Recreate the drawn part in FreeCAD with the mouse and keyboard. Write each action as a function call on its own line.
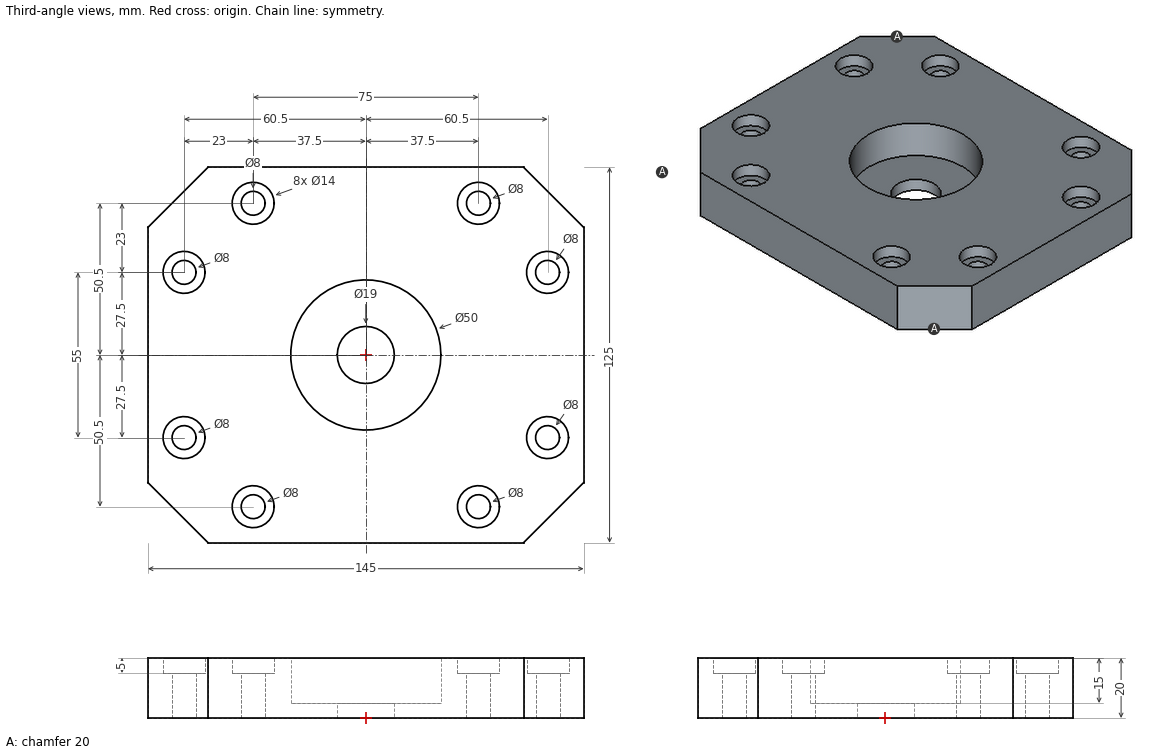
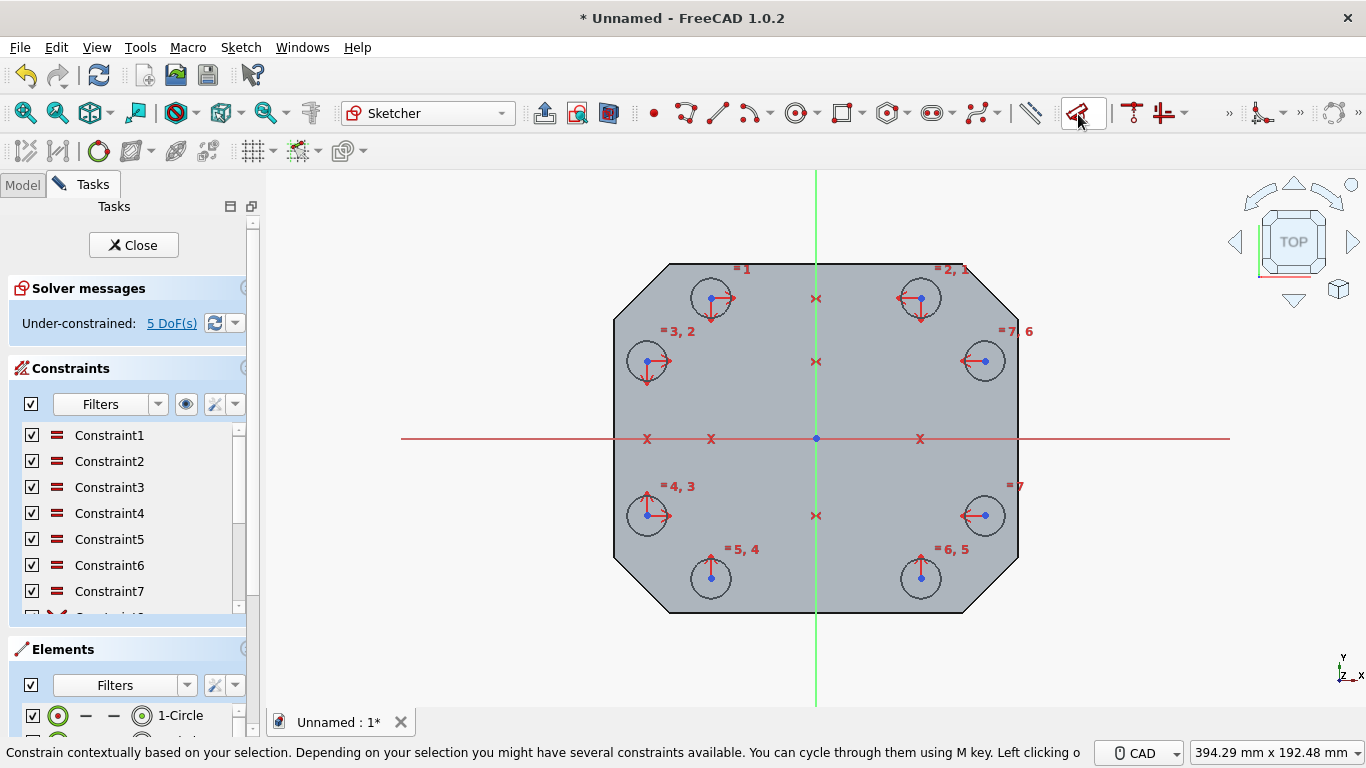
click(725, 284)
click(747, 261)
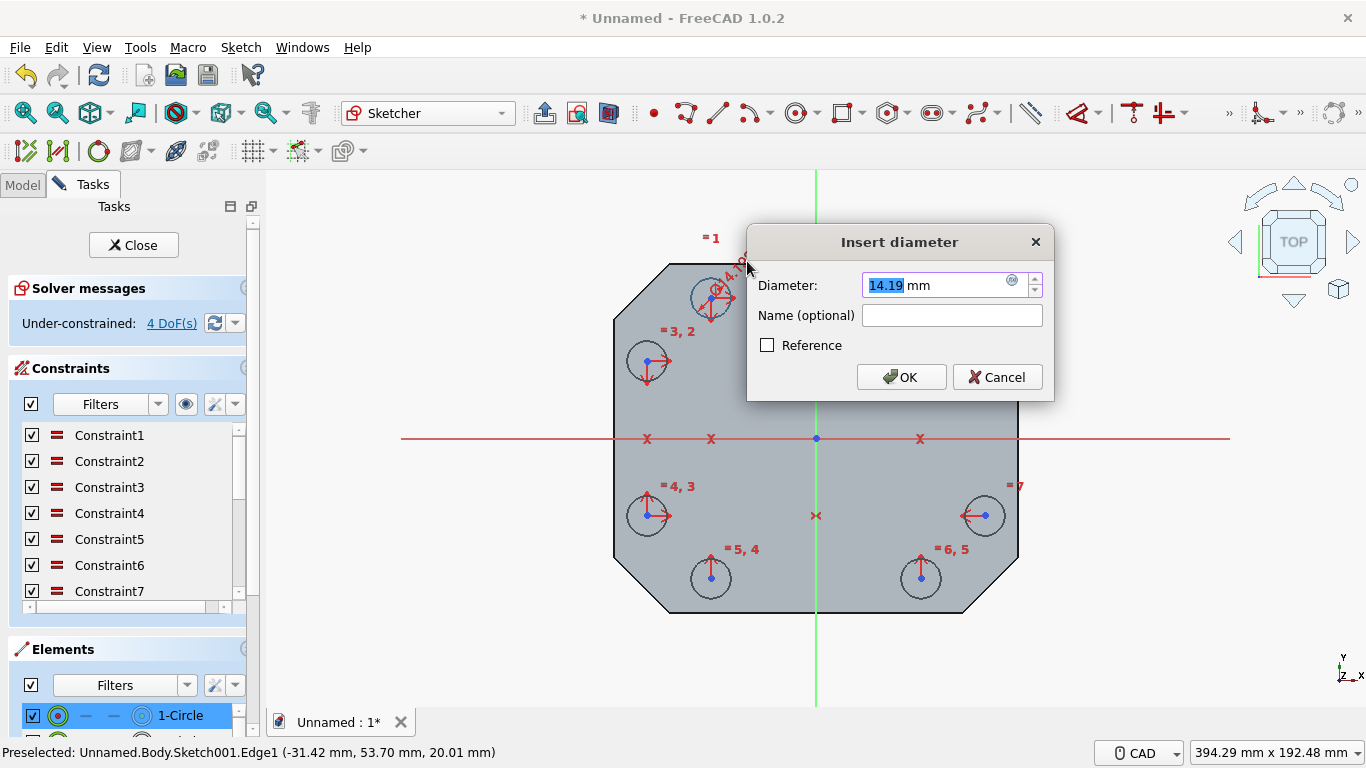
text(14)
key(Return)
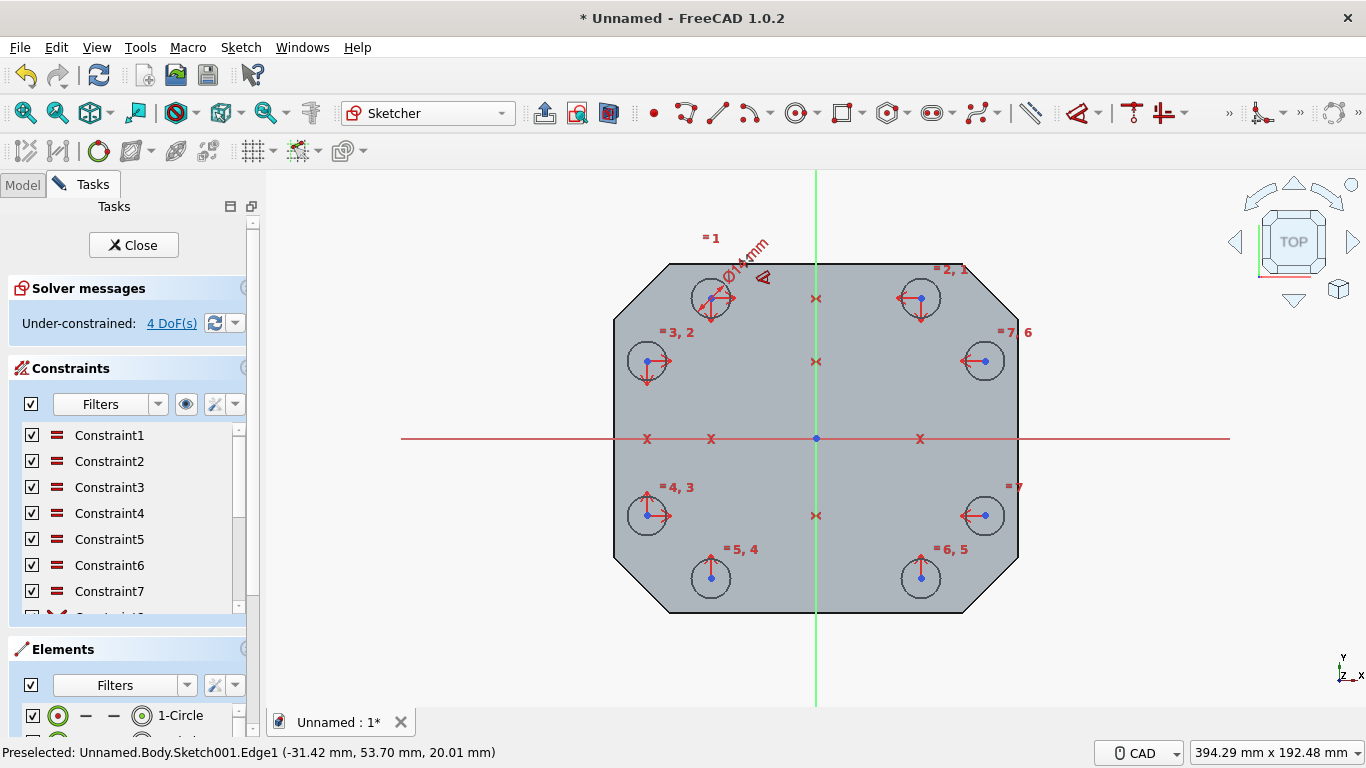
click(711, 298)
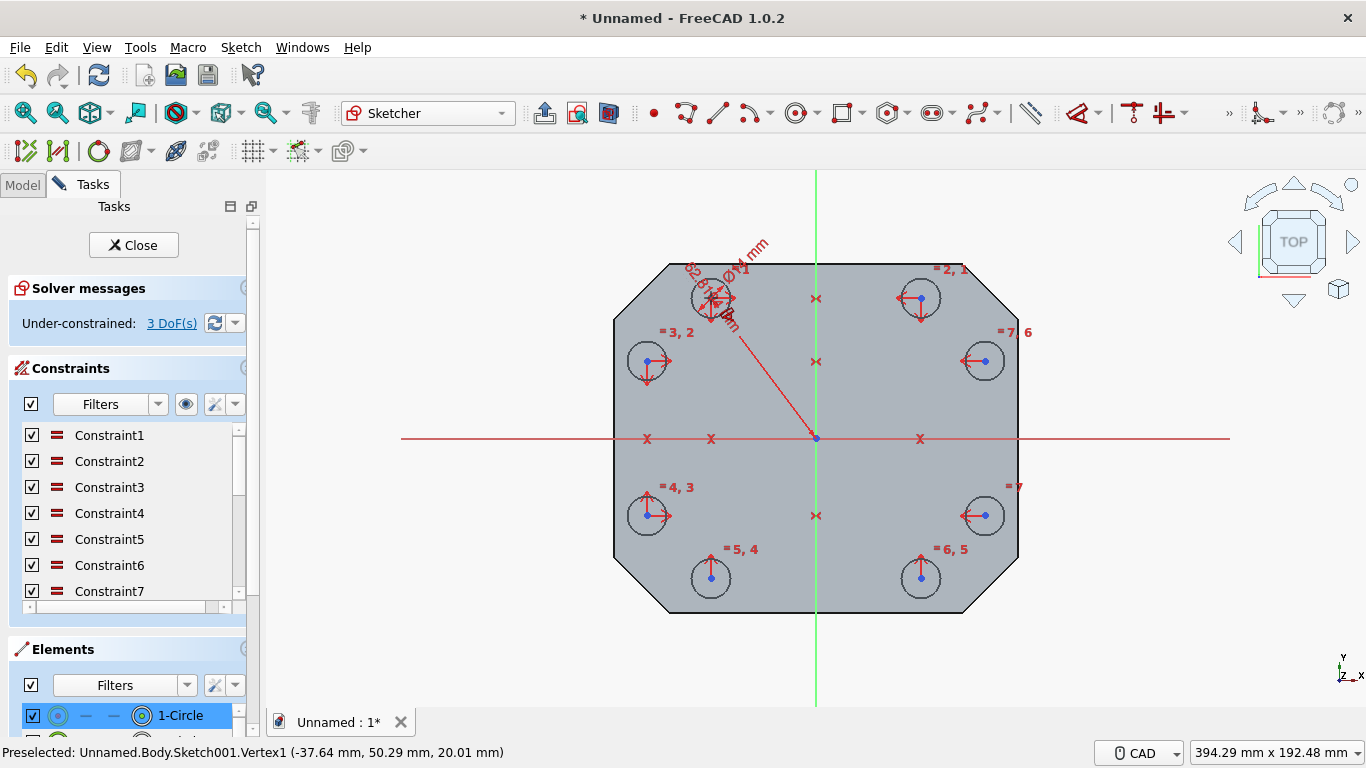
click(921, 298)
click(864, 264)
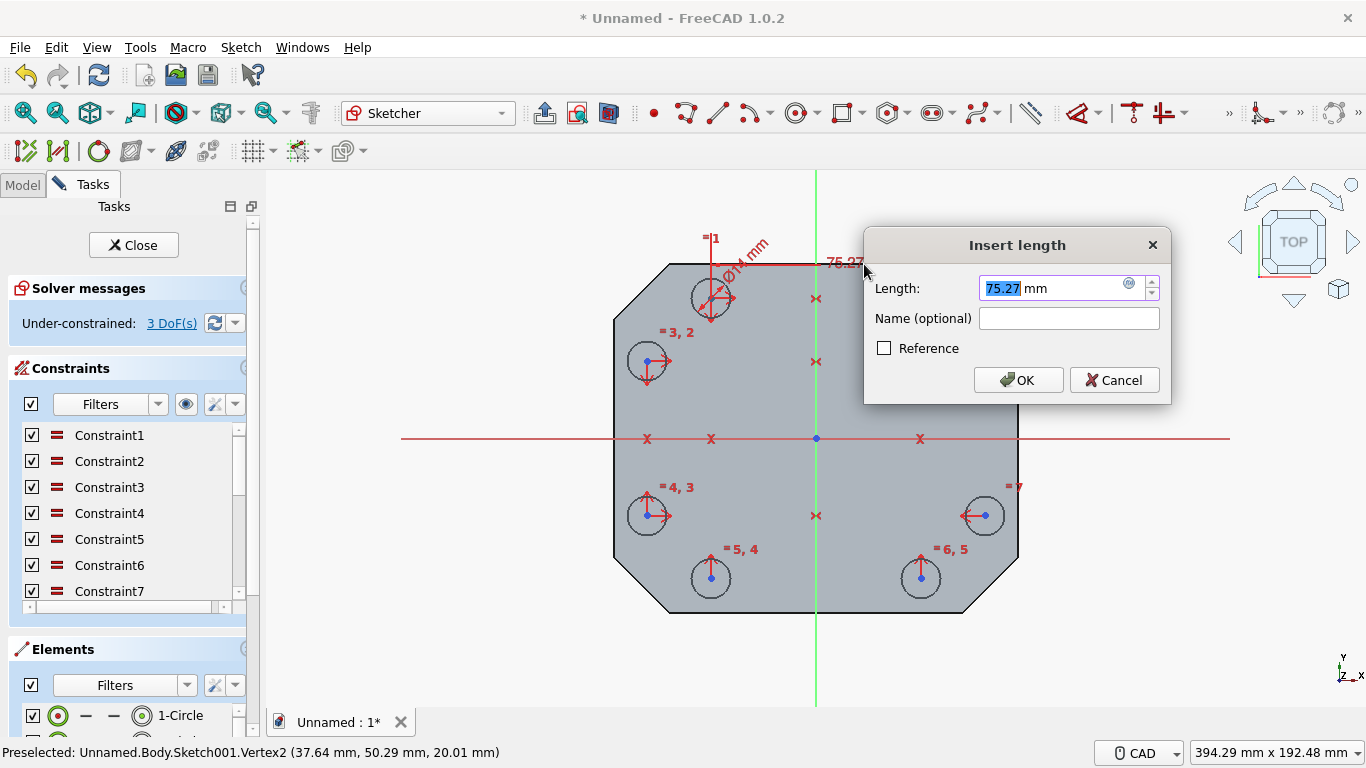
text(75)
key(Return)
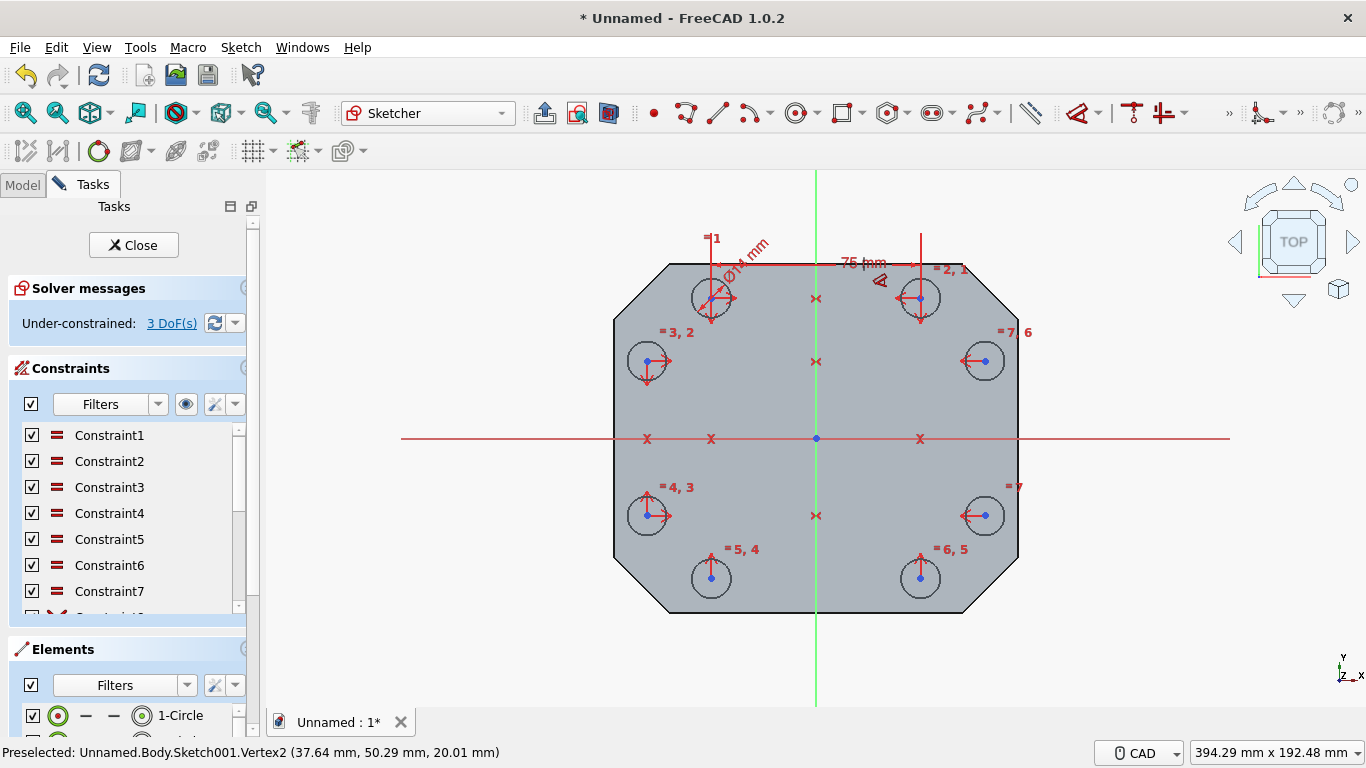
click(711, 298)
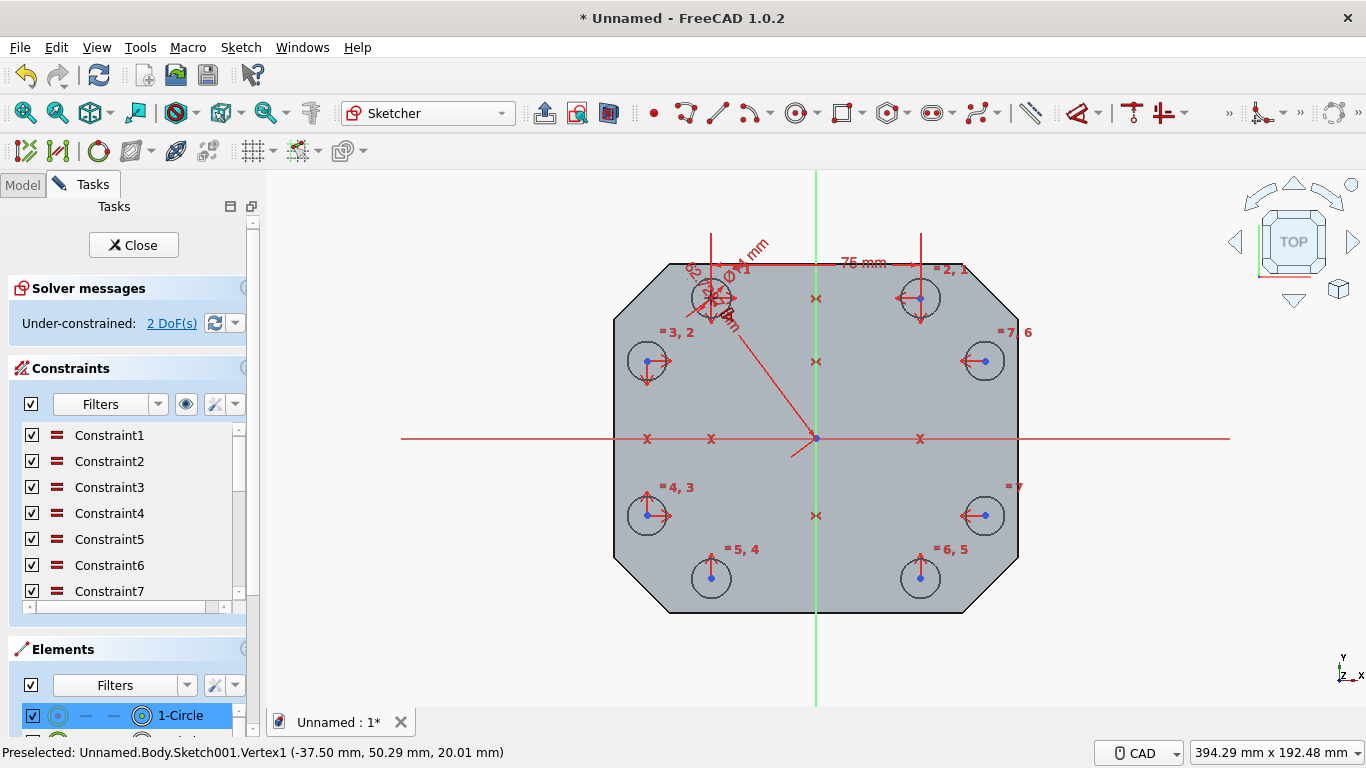
click(647, 361)
click(664, 264)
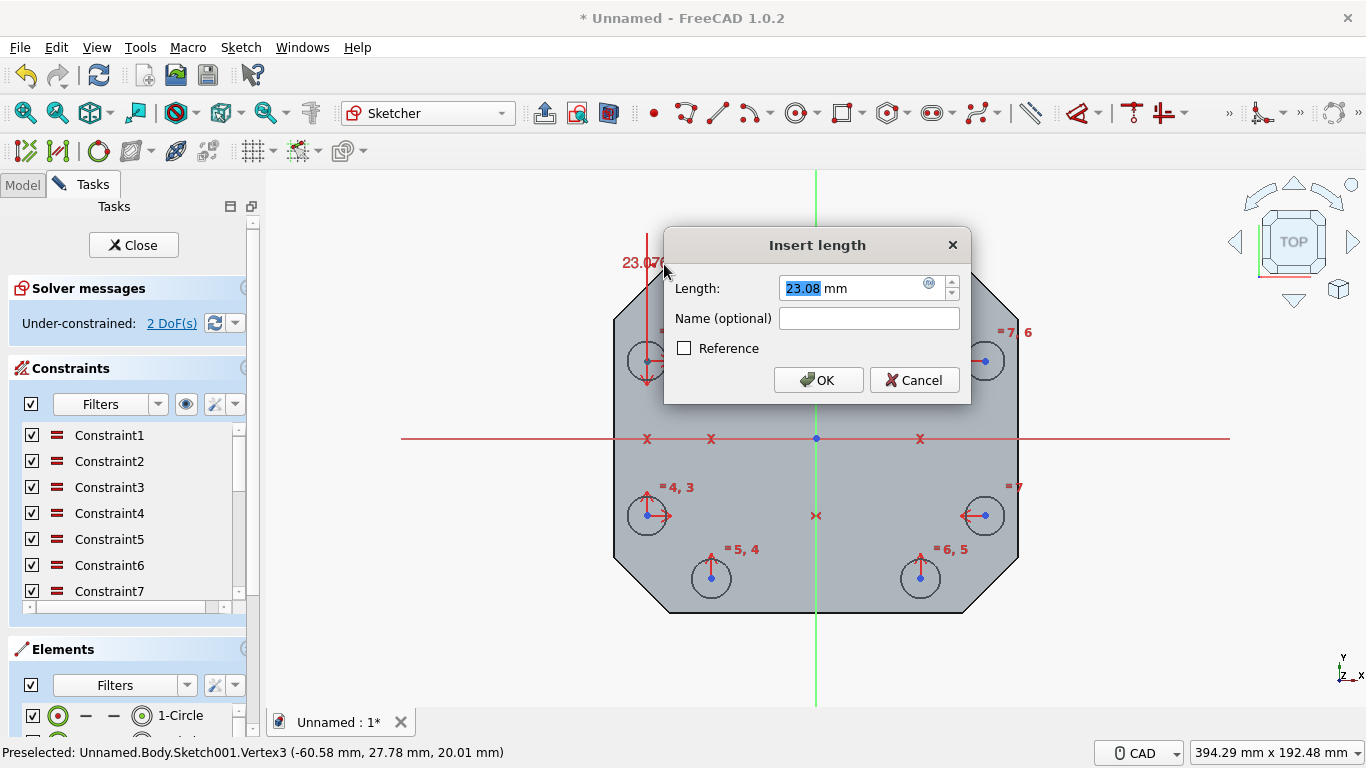
text(23)
key(Return)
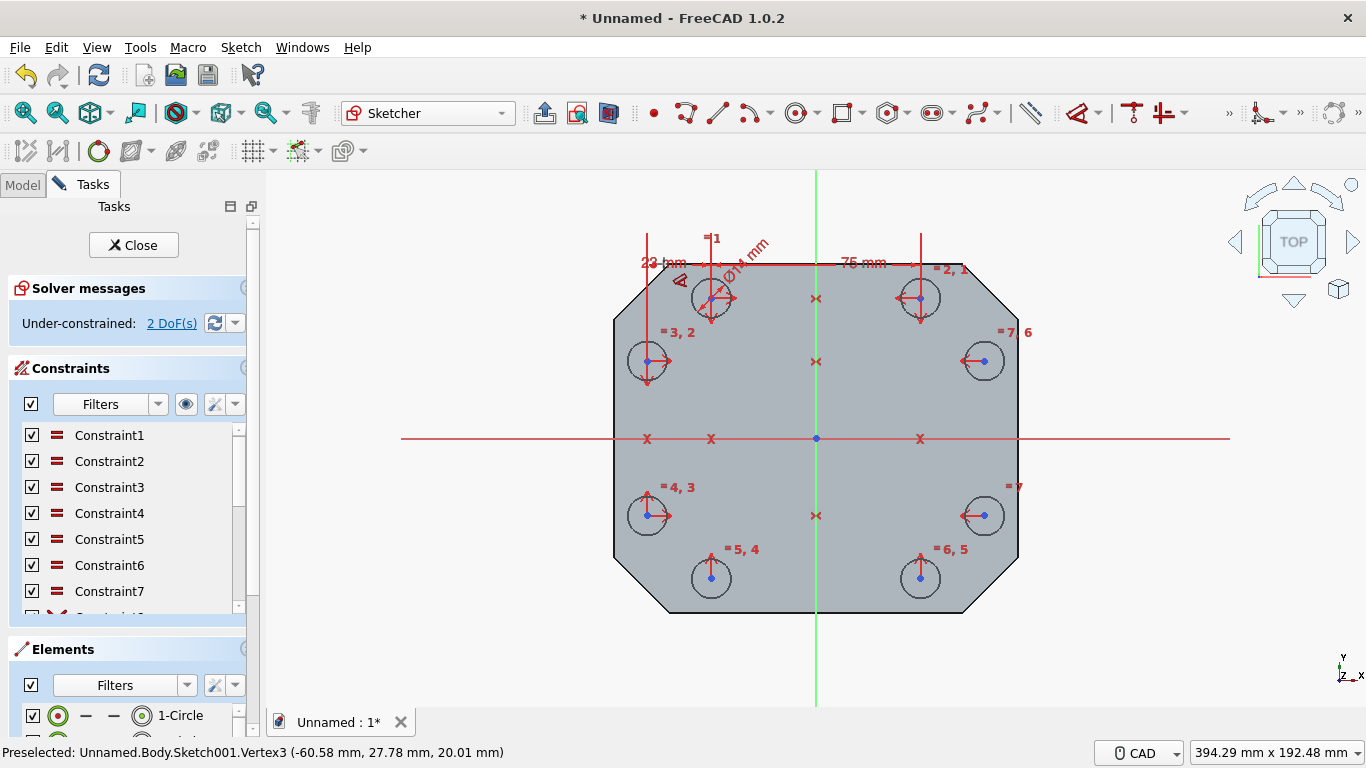
click(711, 298)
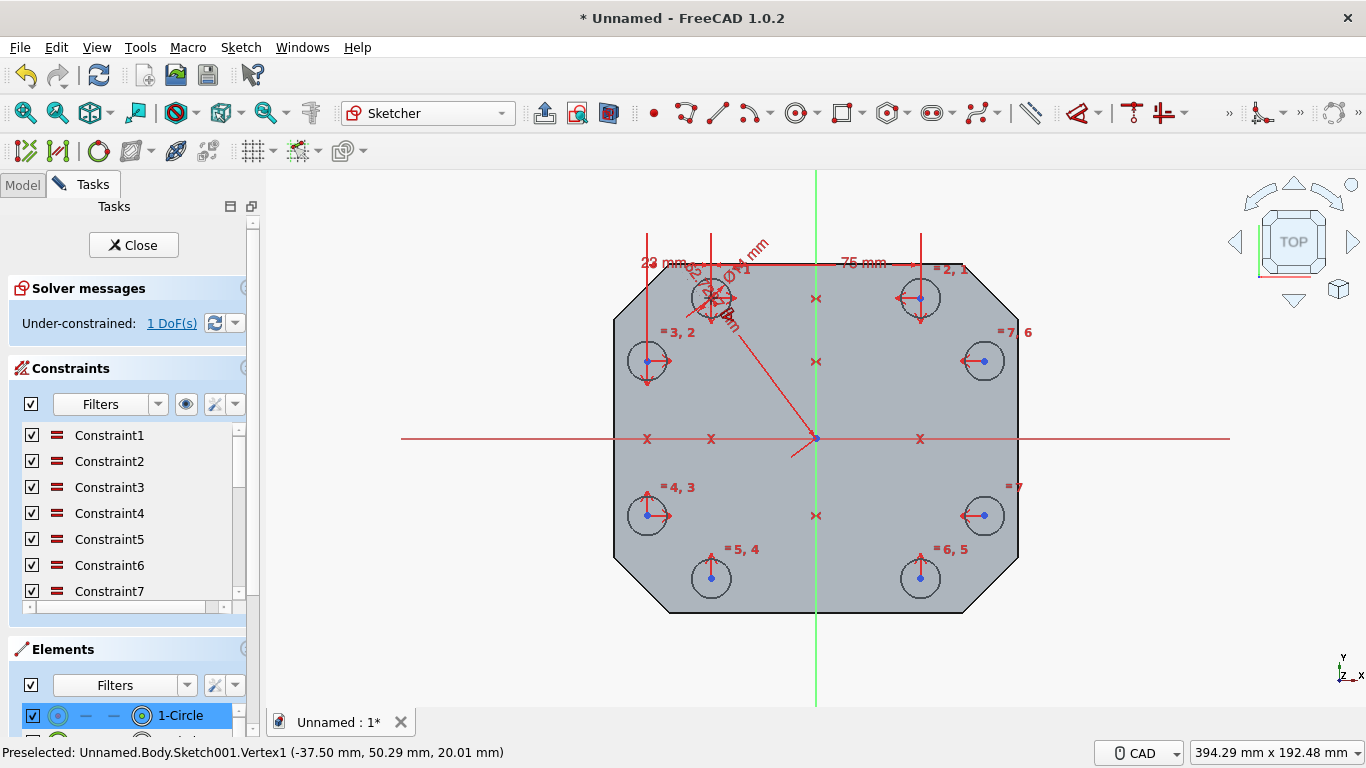
click(647, 361)
click(613, 330)